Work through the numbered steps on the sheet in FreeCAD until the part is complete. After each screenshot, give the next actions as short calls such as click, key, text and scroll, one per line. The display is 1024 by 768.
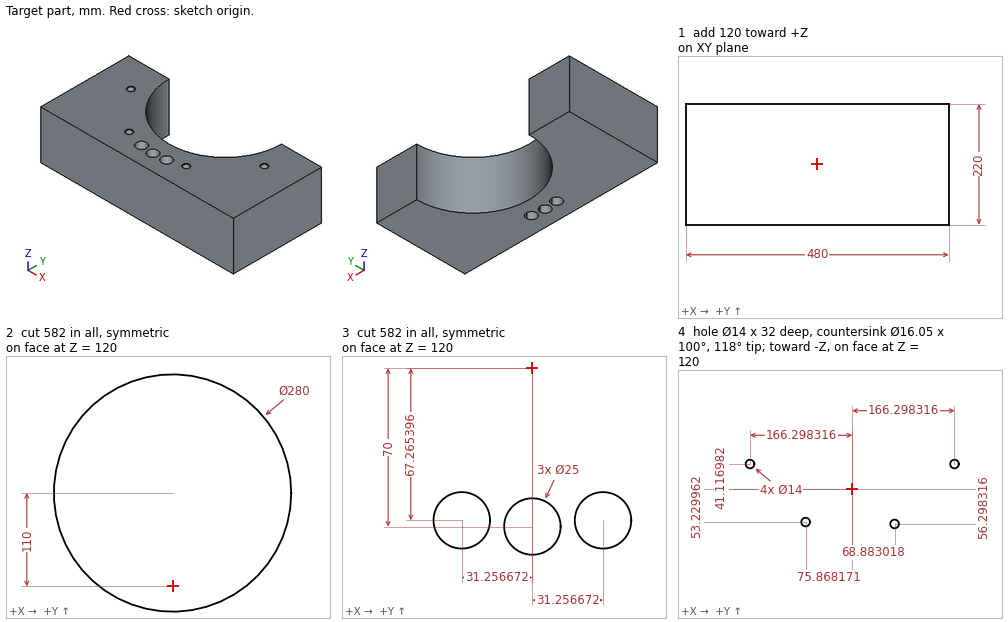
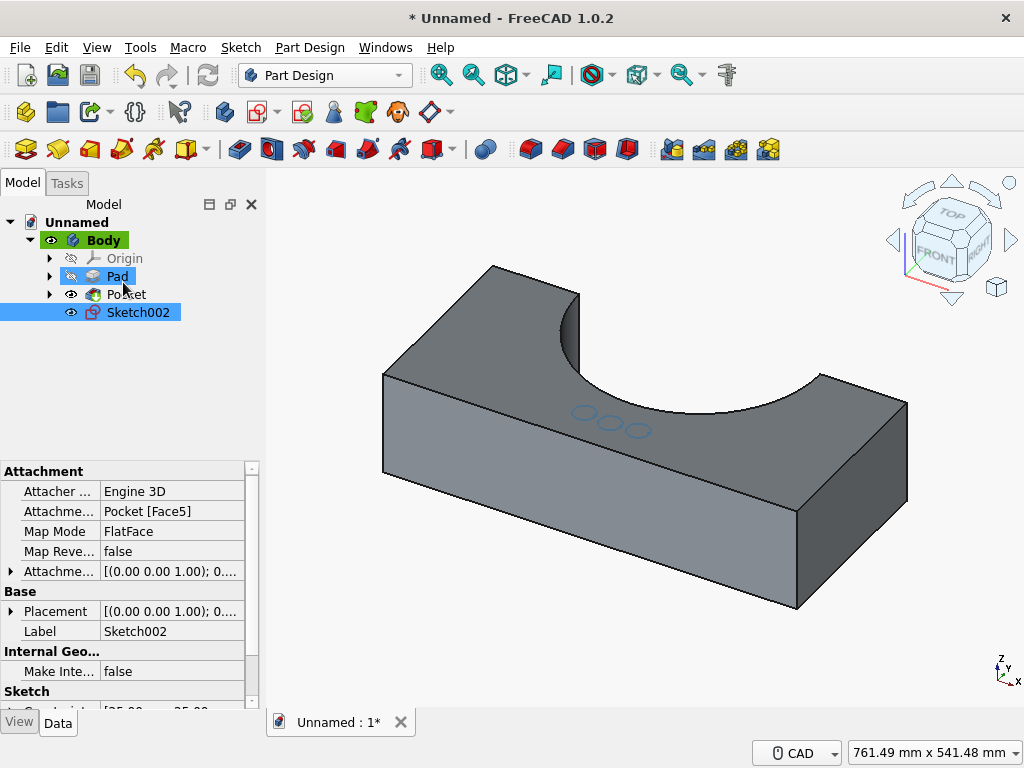
click(240, 150)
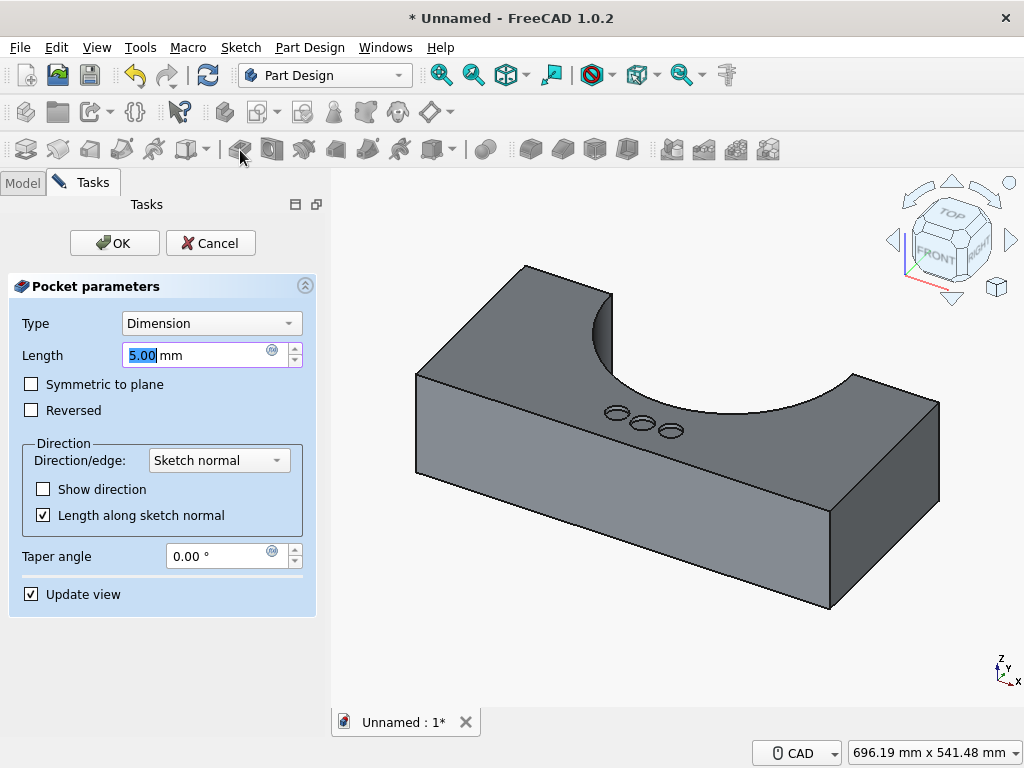
text(582)
key(Tab)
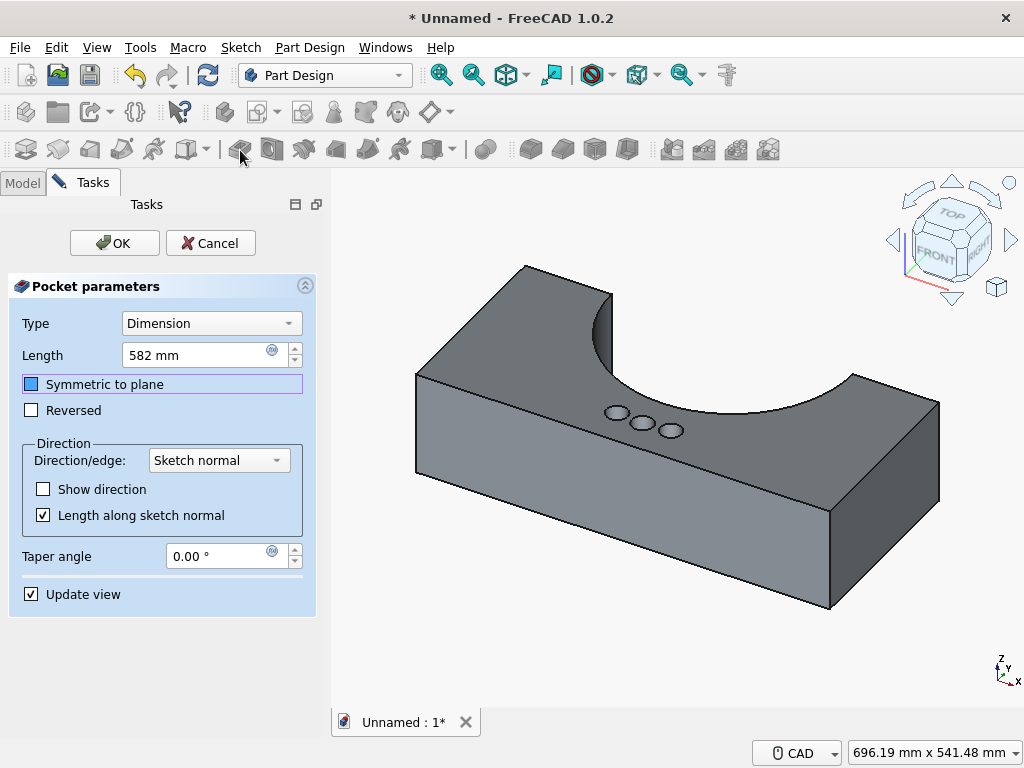
click(30, 384)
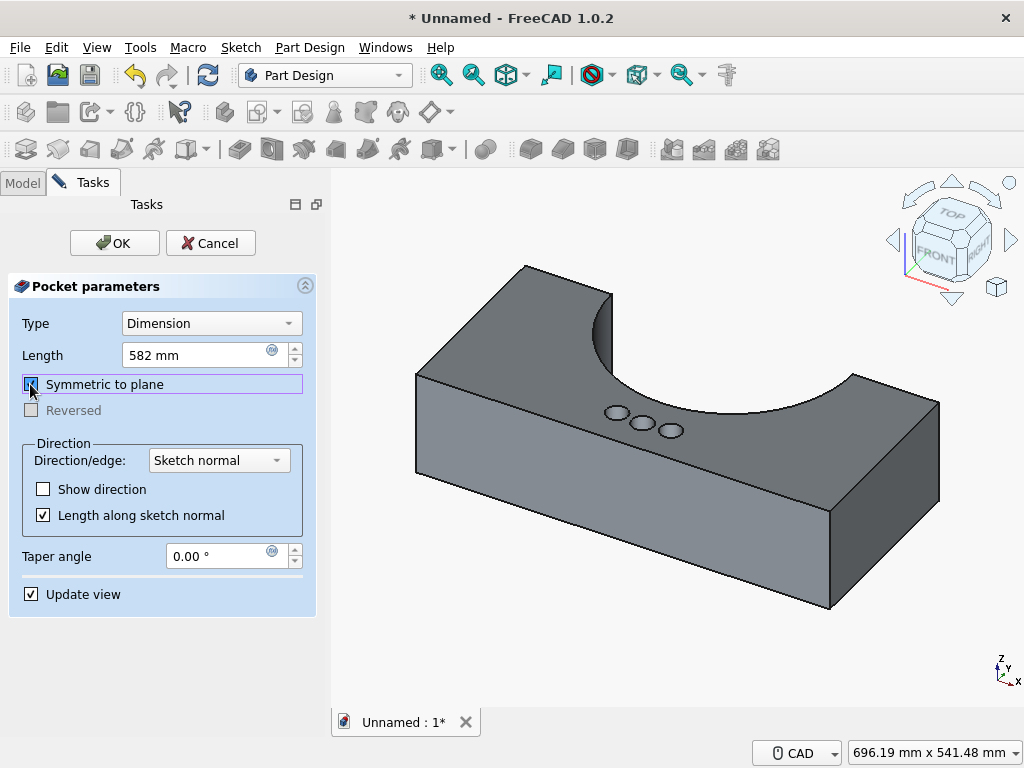
click(115, 243)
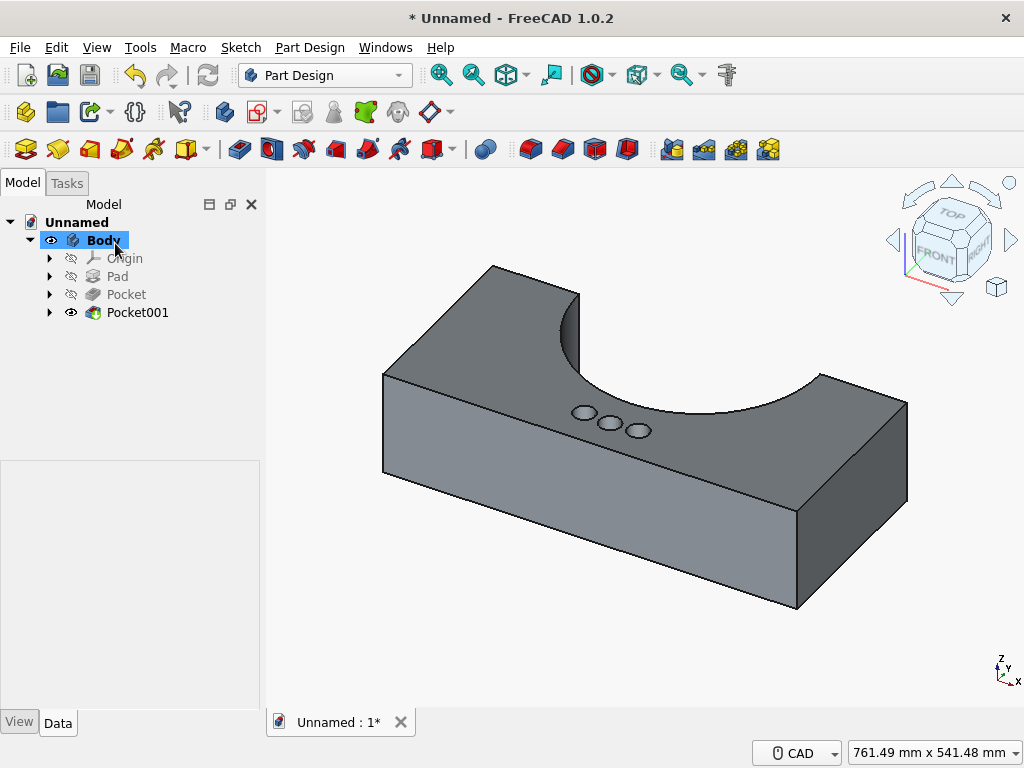
click(748, 442)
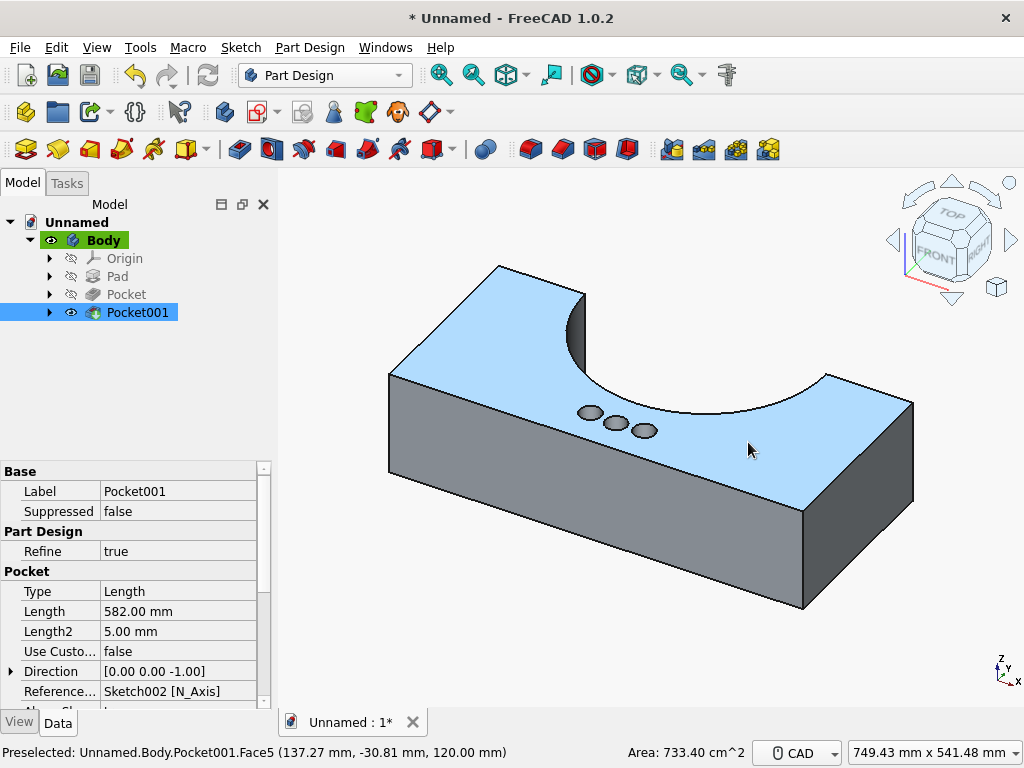
click(258, 112)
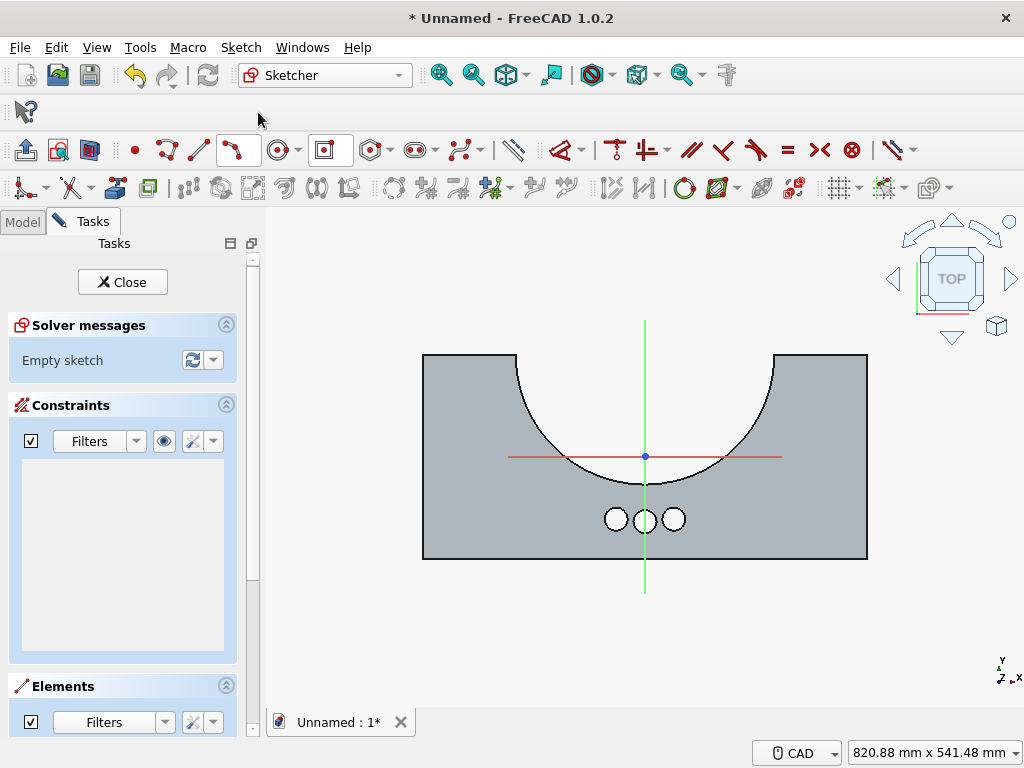
key(g)
key(c)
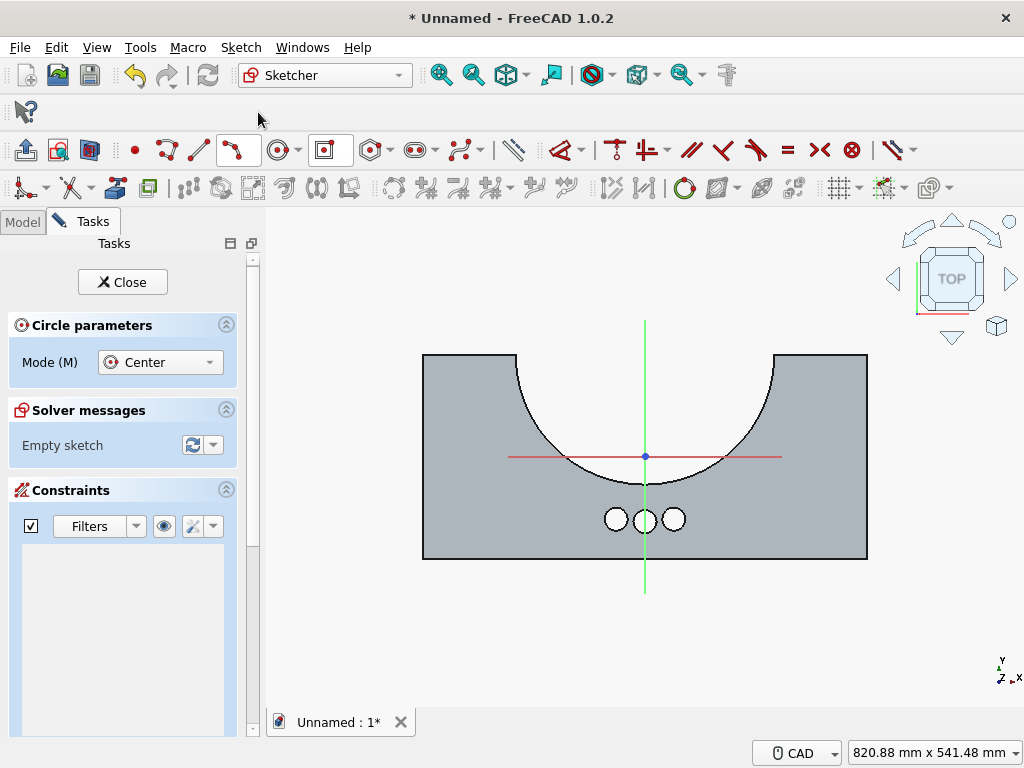
scroll(491, 419, up, 7)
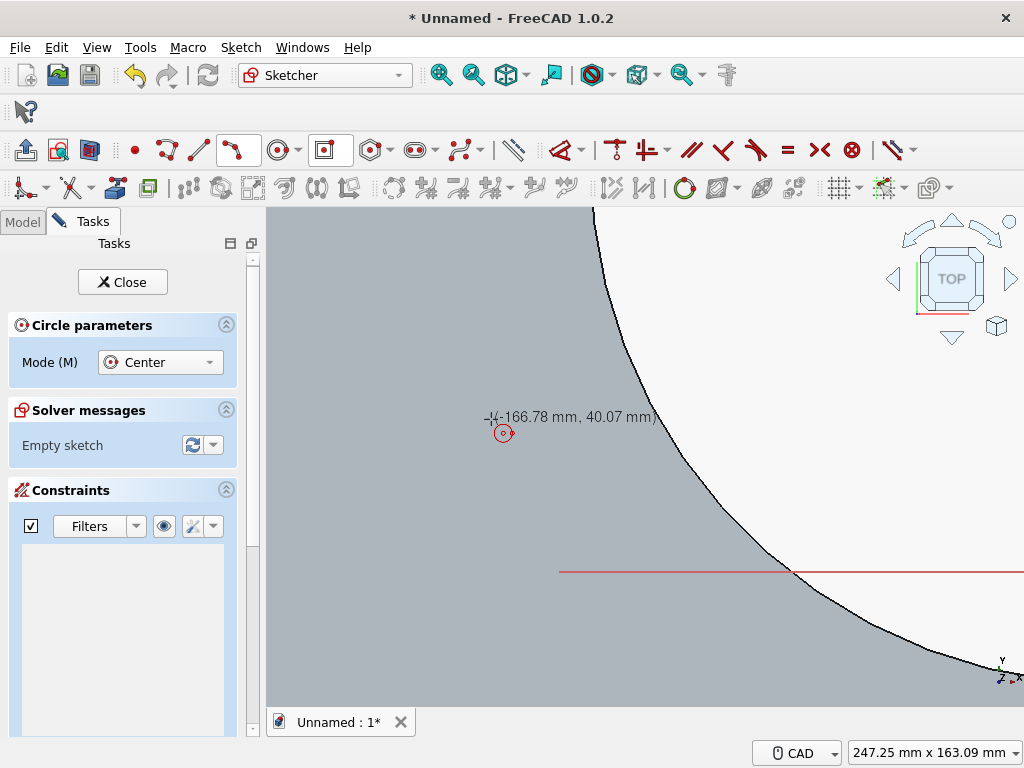
scroll(345, 395, down, 6)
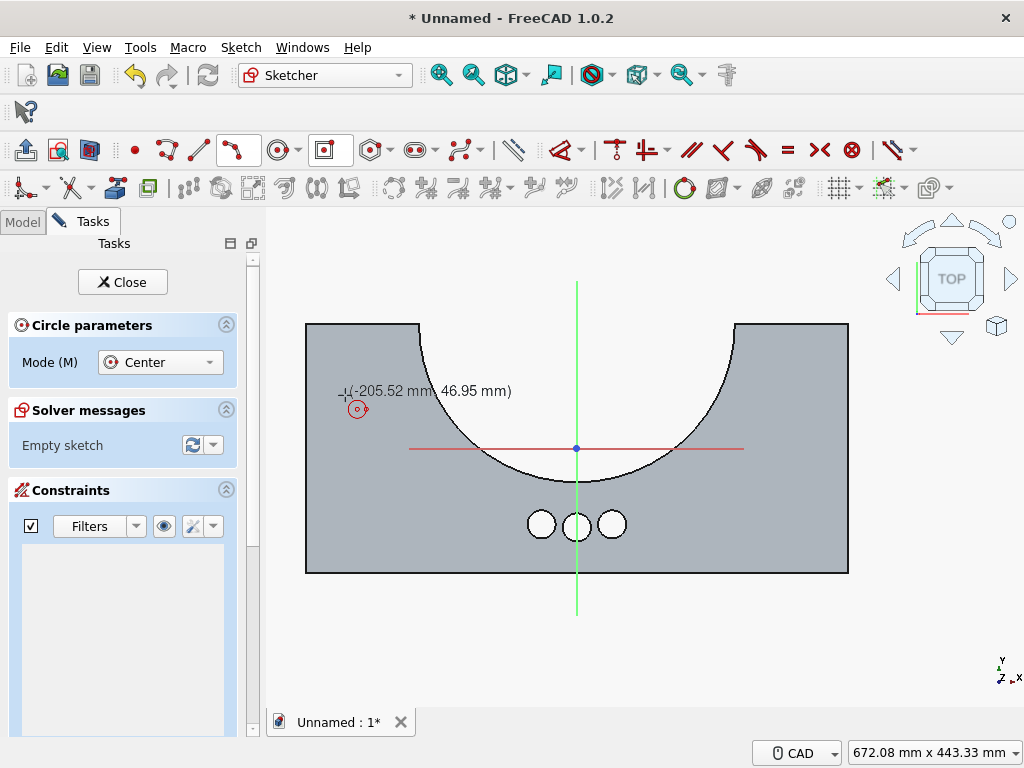
click(389, 402)
move(395, 397)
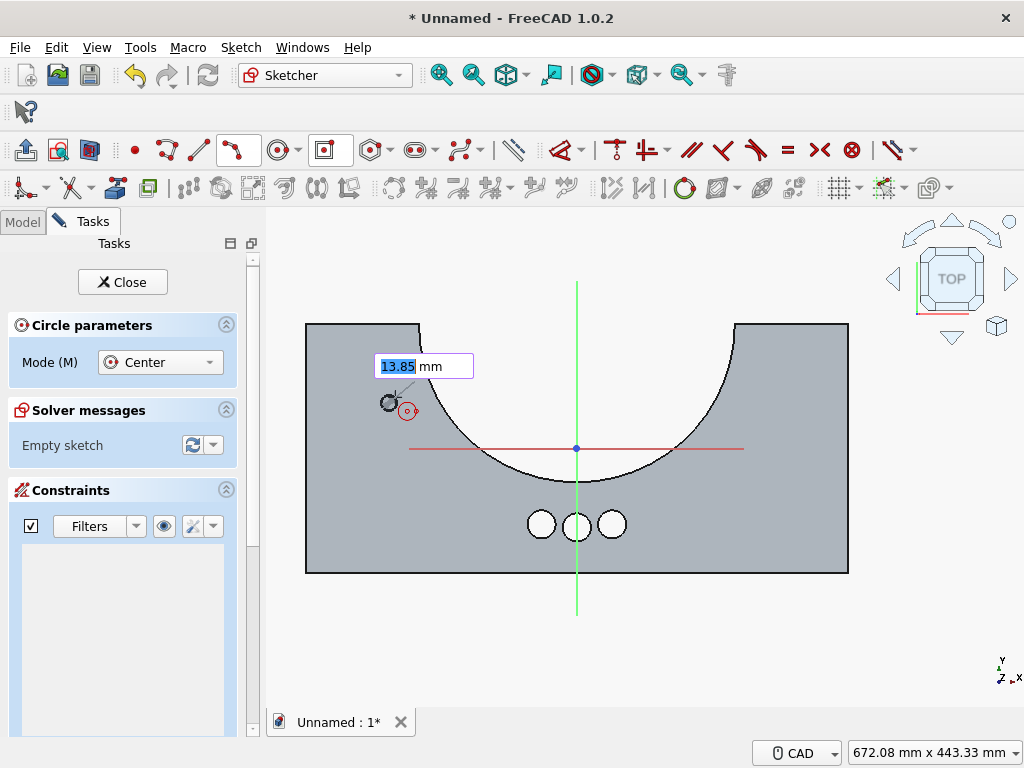
text(14)
key(Return)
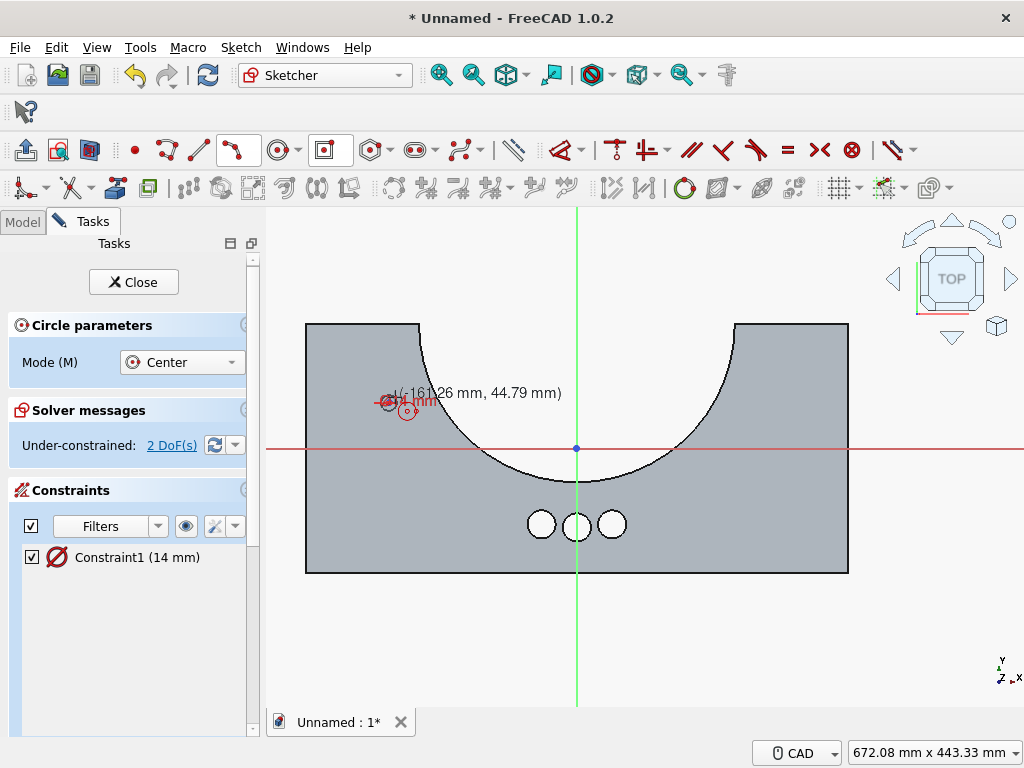
scroll(764, 402, up, 6)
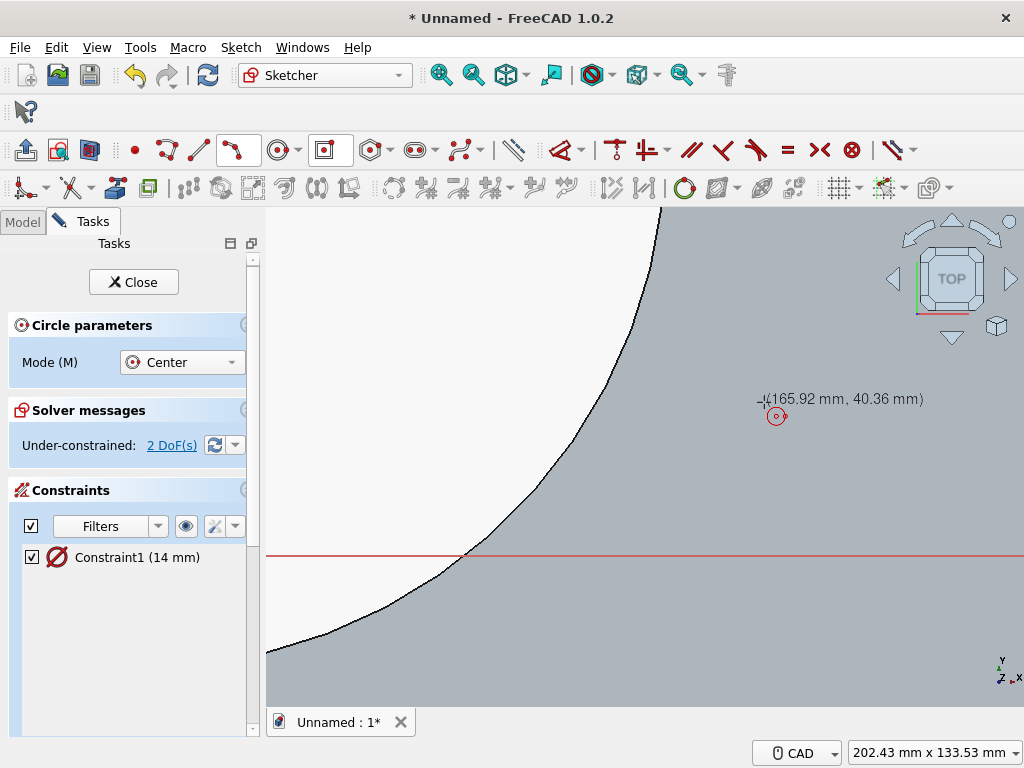
scroll(764, 402, down, 6)